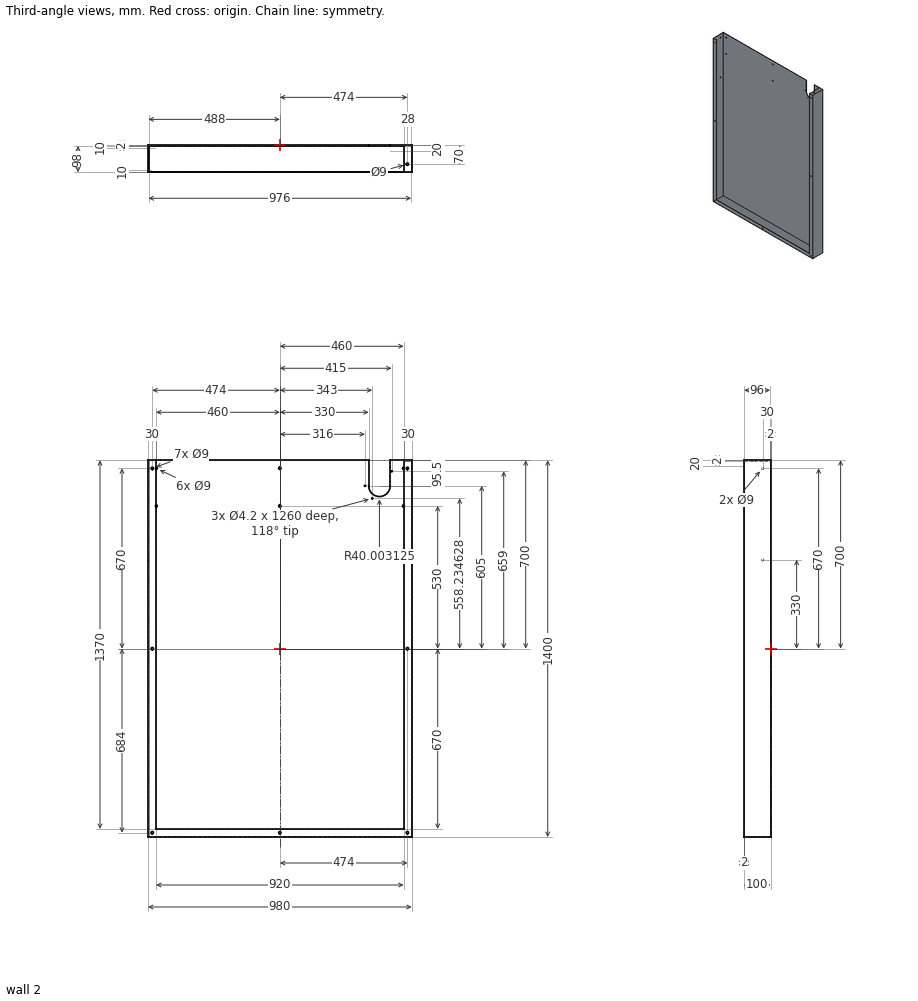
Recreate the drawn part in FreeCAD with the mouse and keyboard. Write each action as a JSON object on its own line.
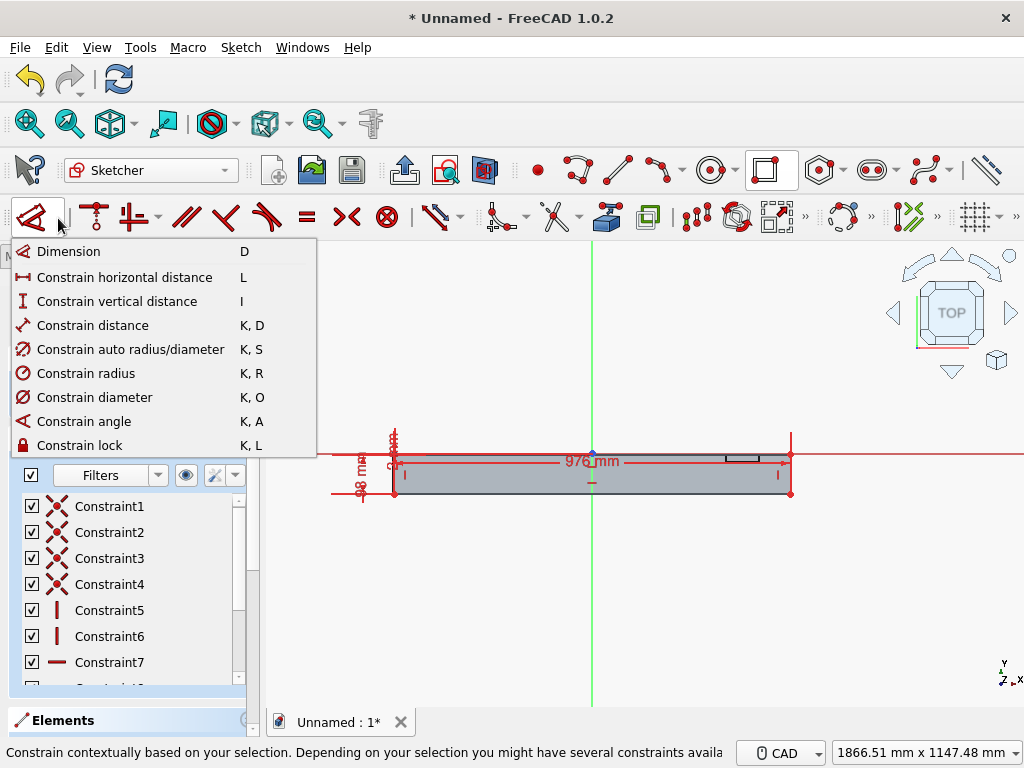
{"action": "left_click", "coordinate": [164, 277]}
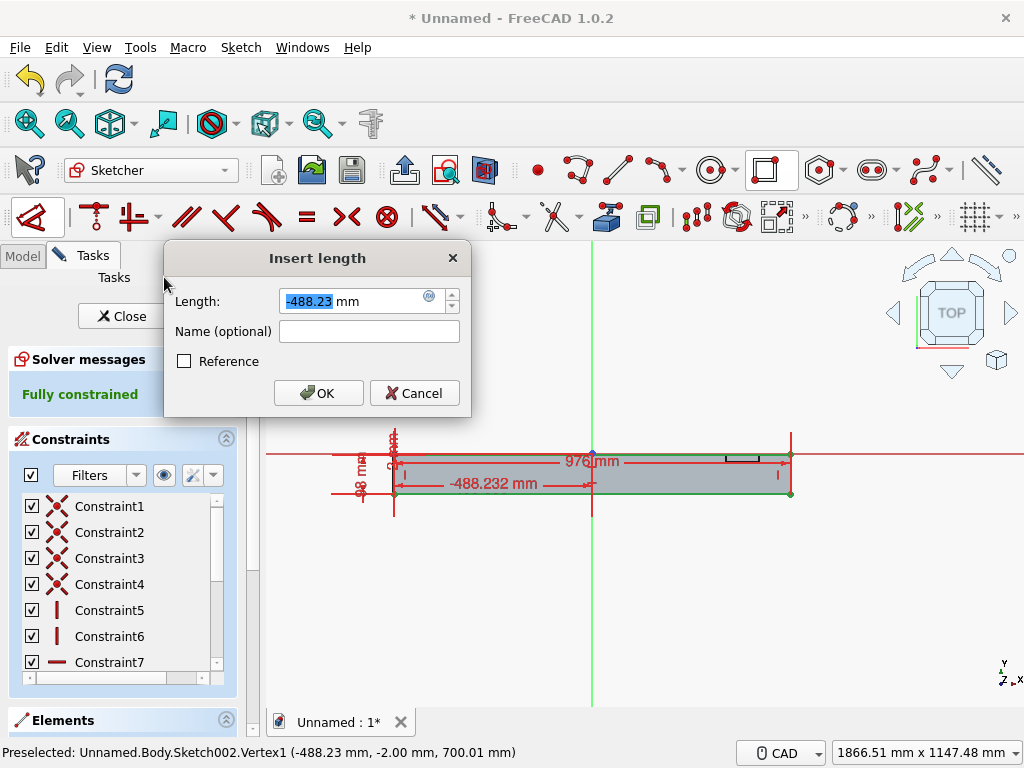
{"action": "type", "text": "-488"}
{"action": "key", "text": "Return"}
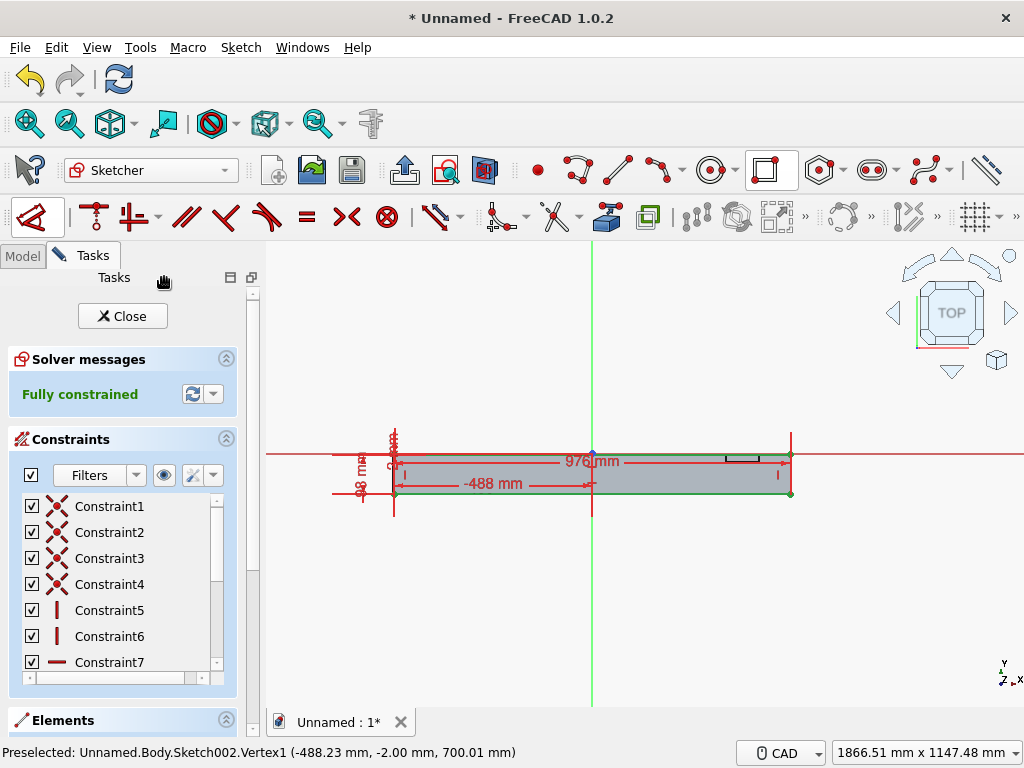
{"action": "left_click", "coordinate": [123, 316]}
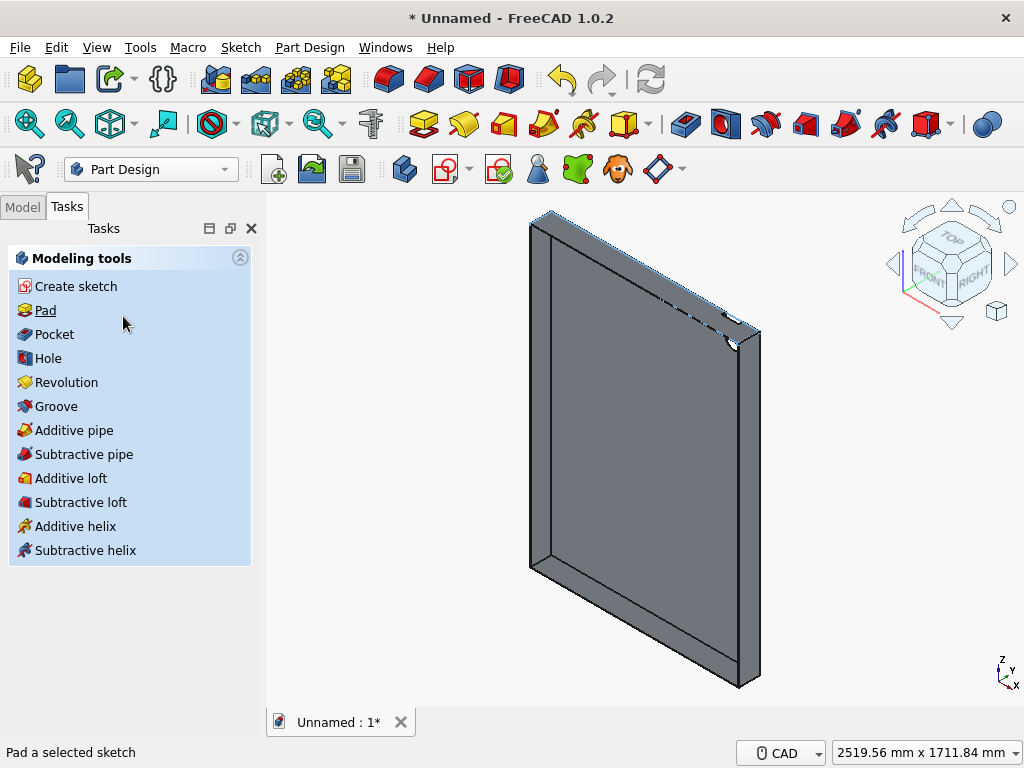
{"action": "left_click", "coordinate": [686, 124]}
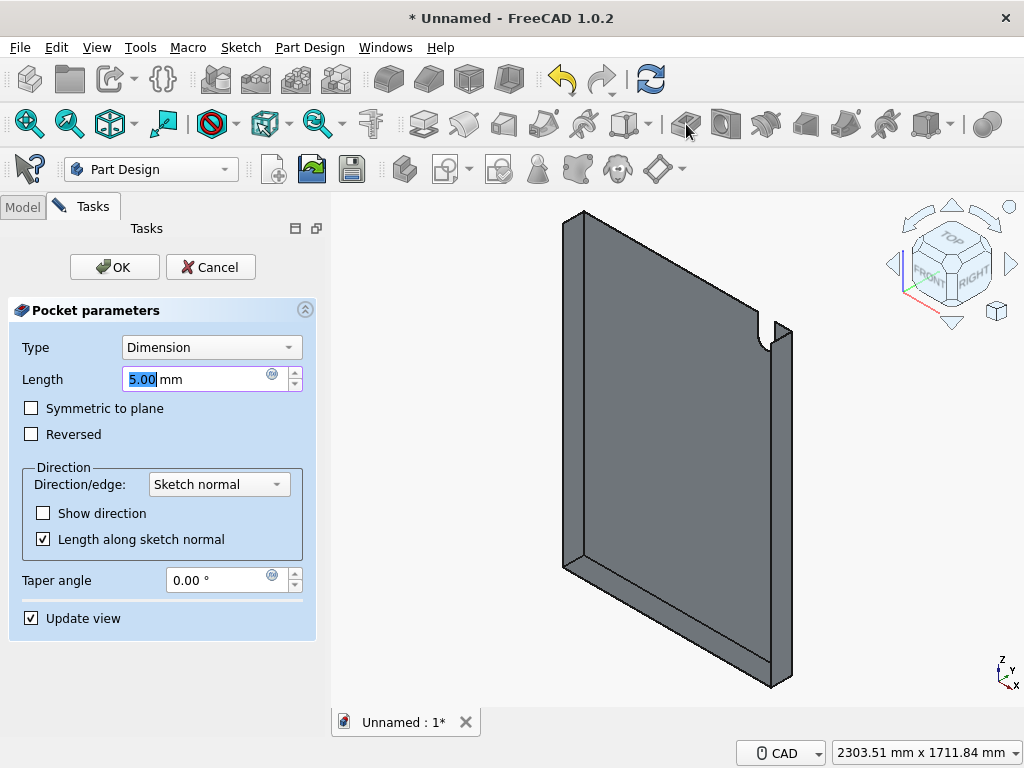
{"action": "type", "text": "20"}
{"action": "key", "text": "Tab"}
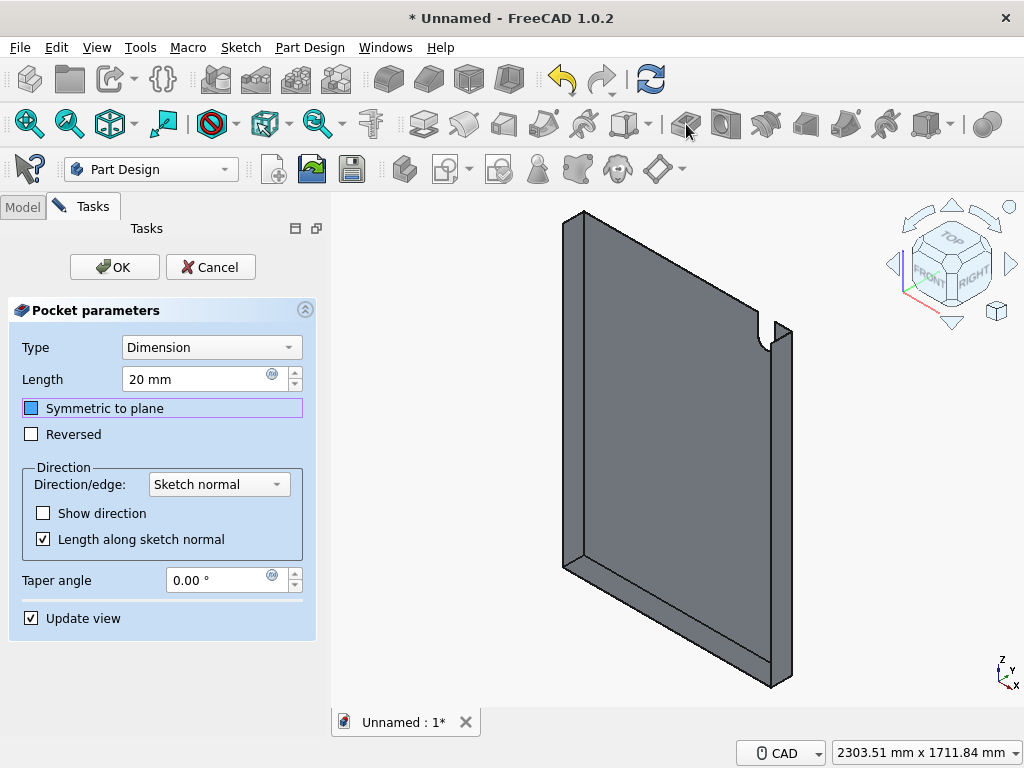
{"action": "left_click", "coordinate": [115, 267]}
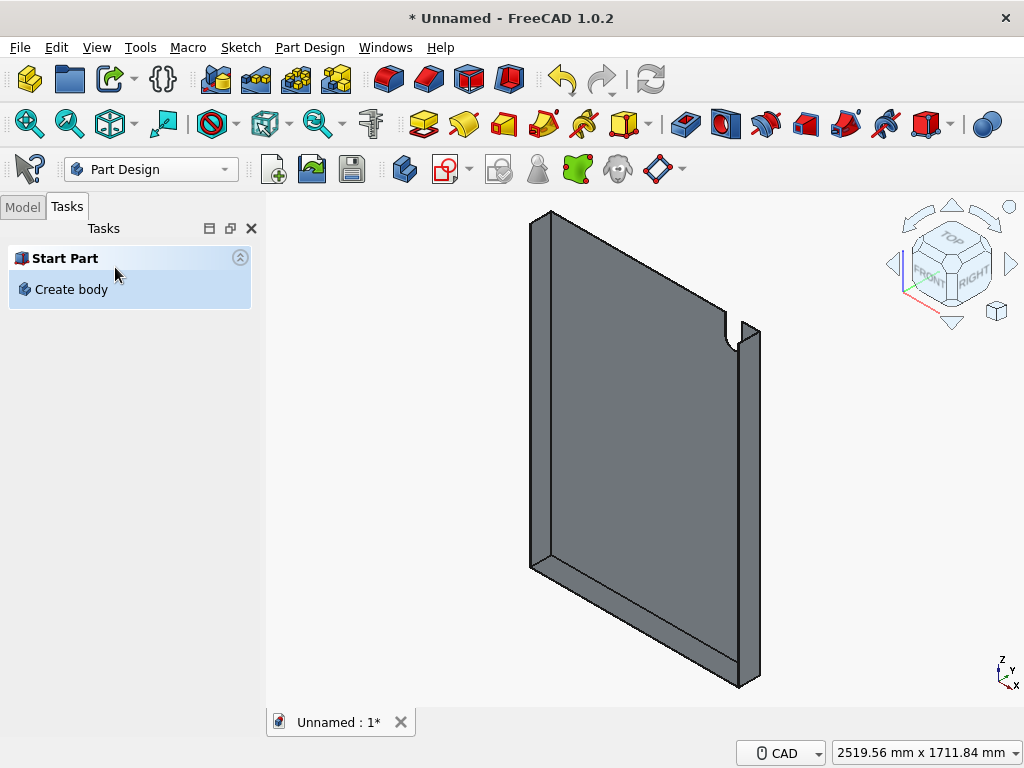
{"action": "scroll", "coordinate": [738, 457], "scroll_direction": "up", "scroll_amount": 15}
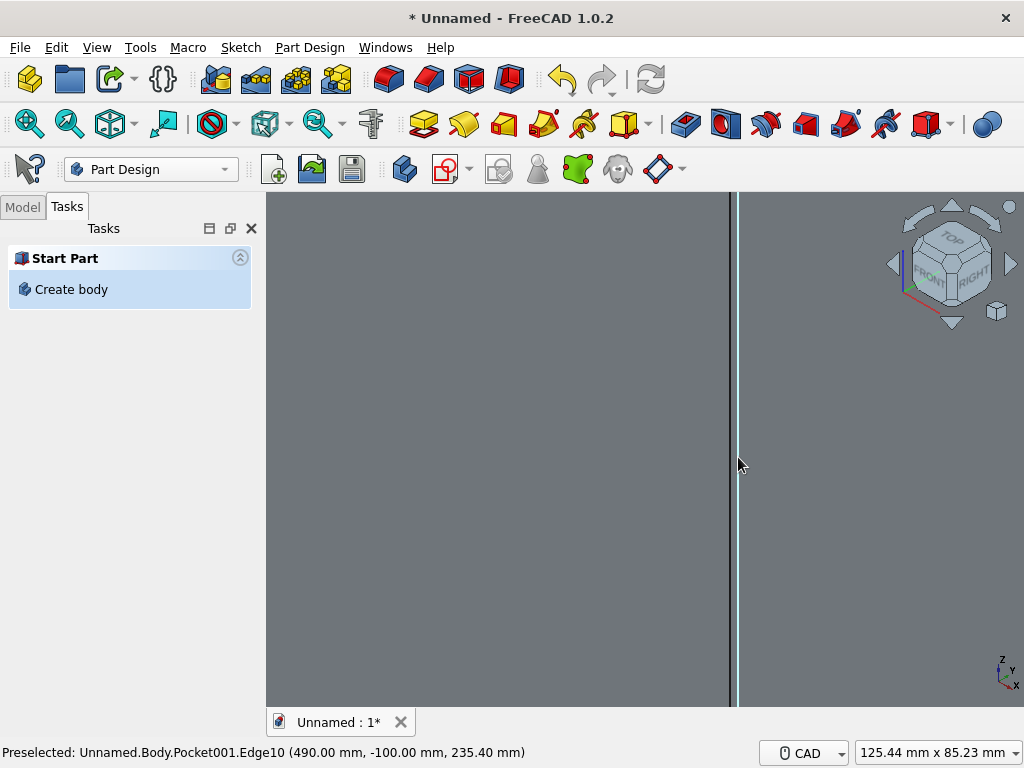
{"action": "scroll", "coordinate": [732, 470], "scroll_direction": "up", "scroll_amount": 6}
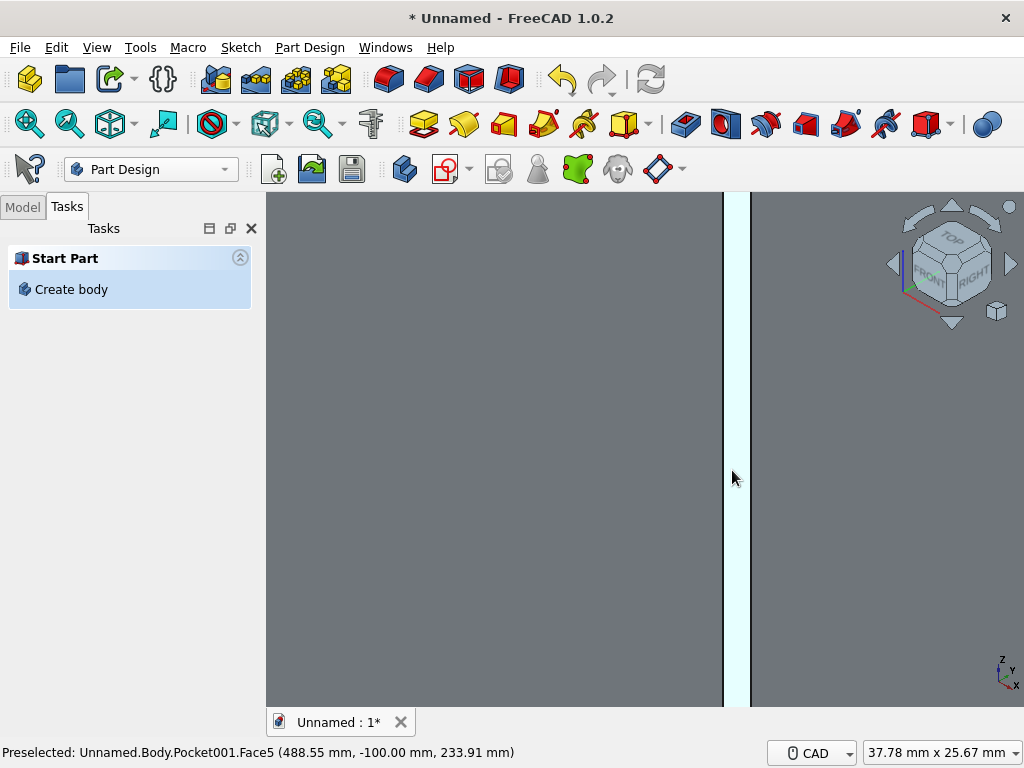
{"action": "left_click", "coordinate": [732, 471]}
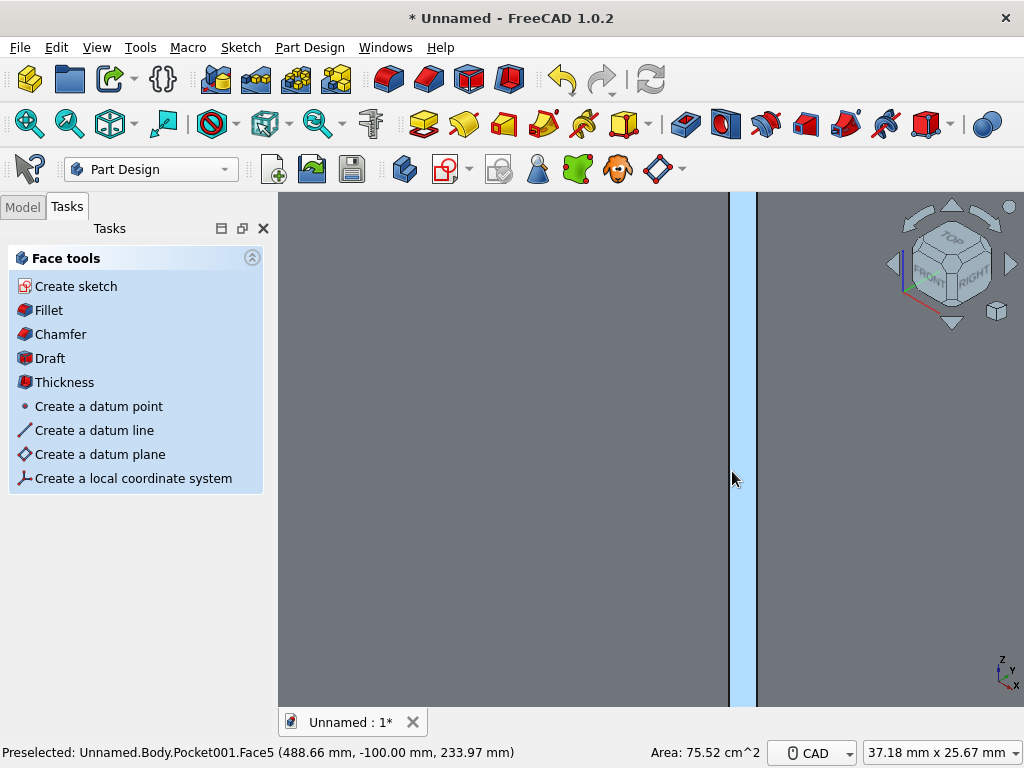
{"action": "left_click", "coordinate": [446, 170]}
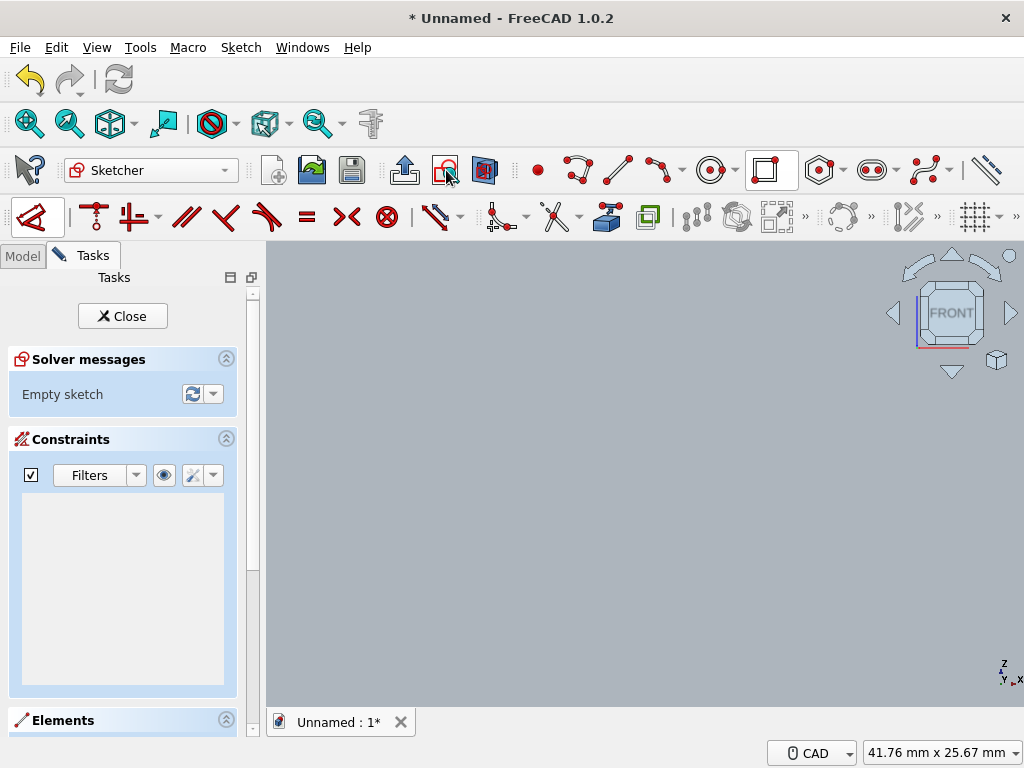
{"action": "scroll", "coordinate": [576, 474], "scroll_direction": "down", "scroll_amount": 15}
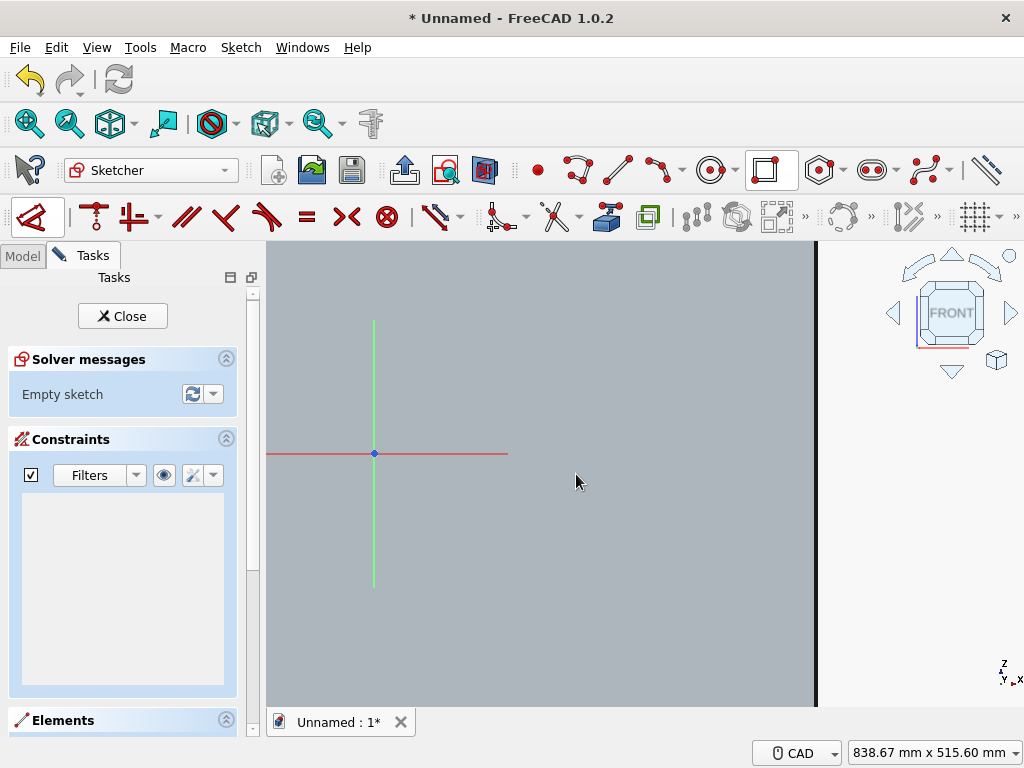
{"action": "scroll", "coordinate": [643, 481], "scroll_direction": "down", "scroll_amount": 7}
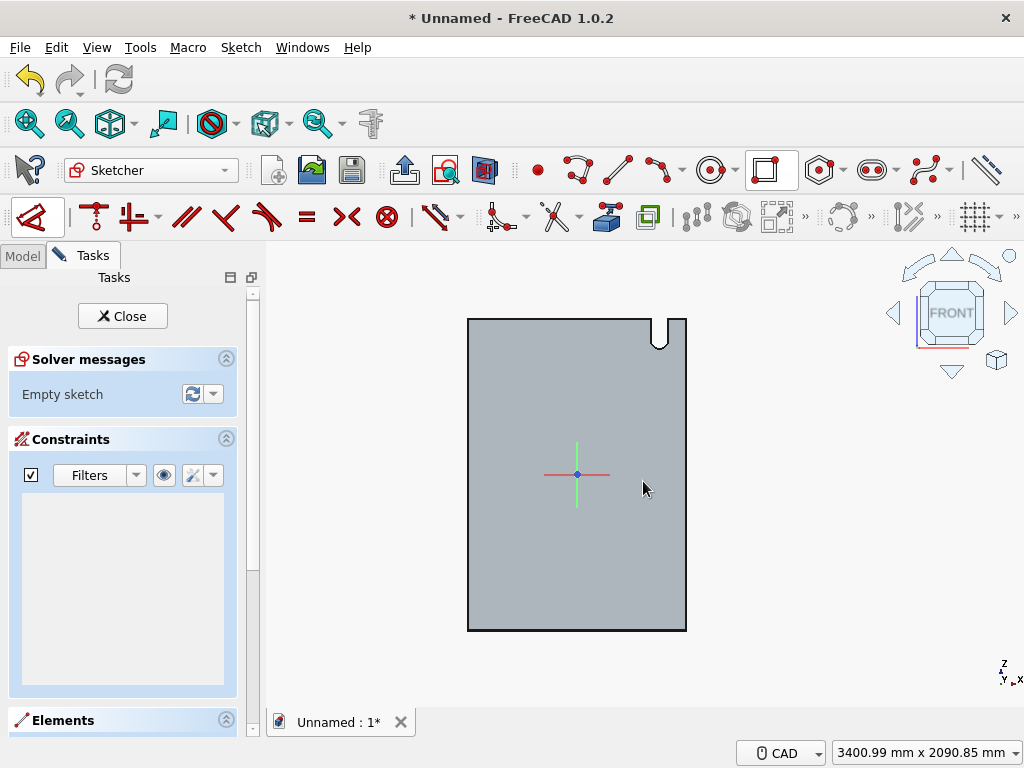
{"action": "left_click", "coordinate": [578, 170]}